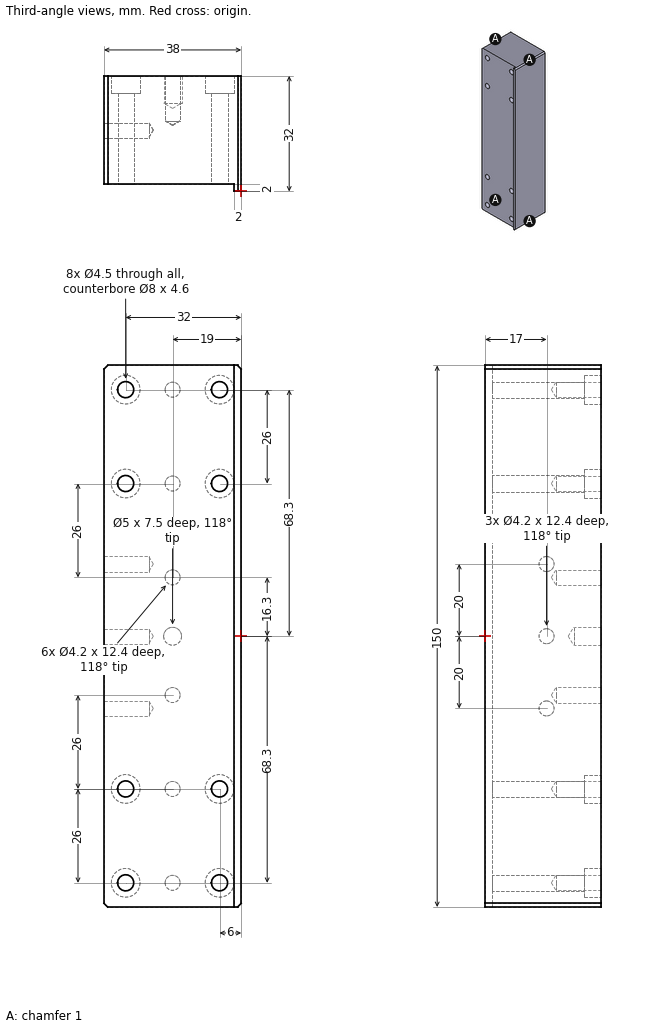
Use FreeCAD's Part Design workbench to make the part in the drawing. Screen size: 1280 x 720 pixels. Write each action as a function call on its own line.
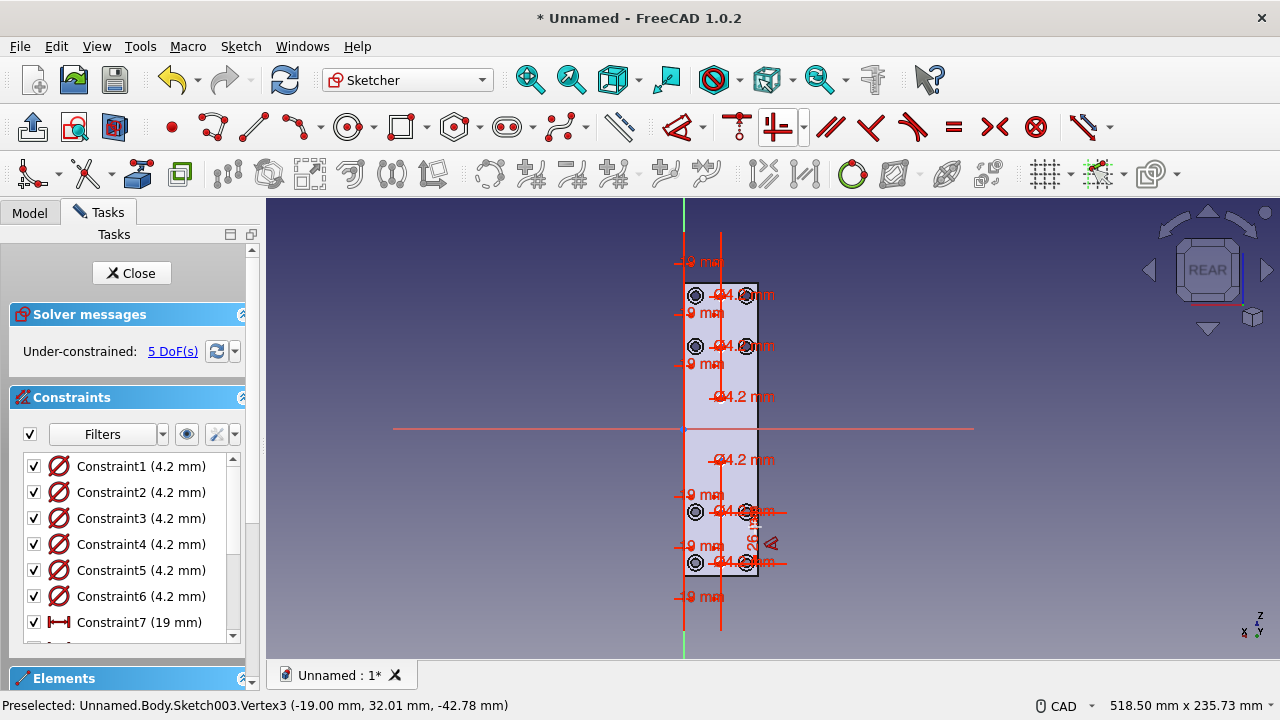
click(721, 399)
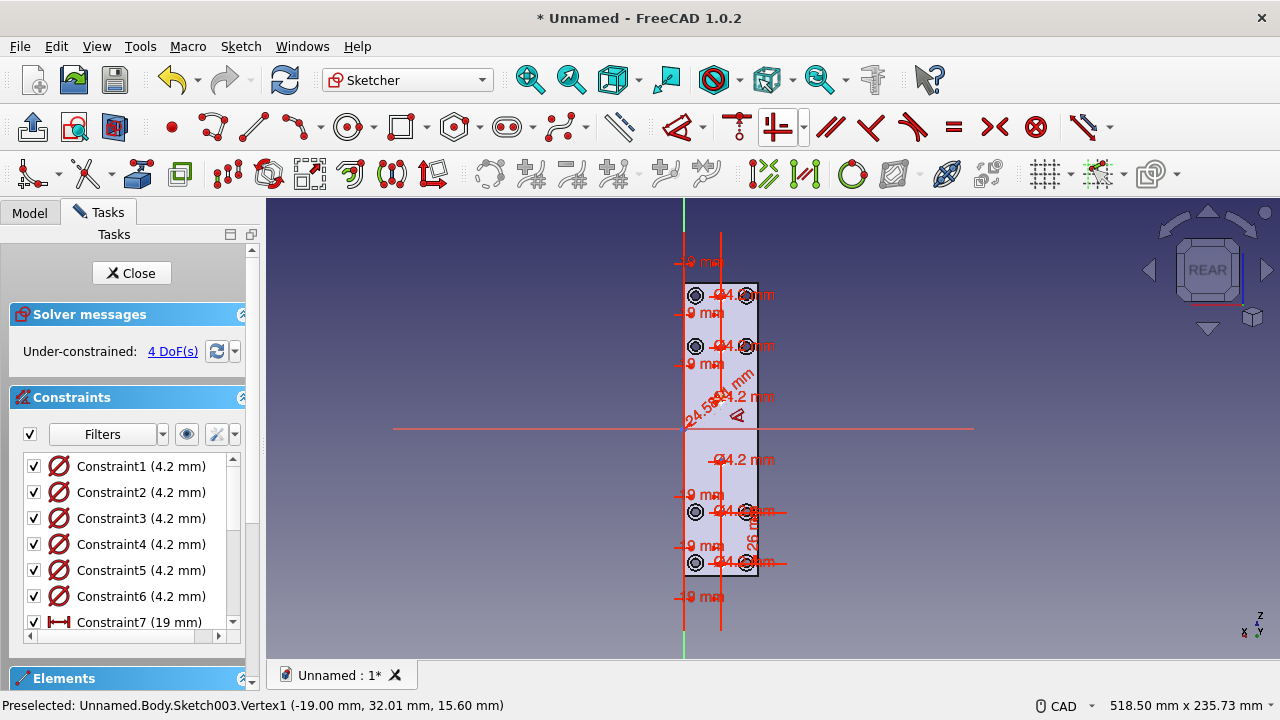
click(721, 348)
click(755, 385)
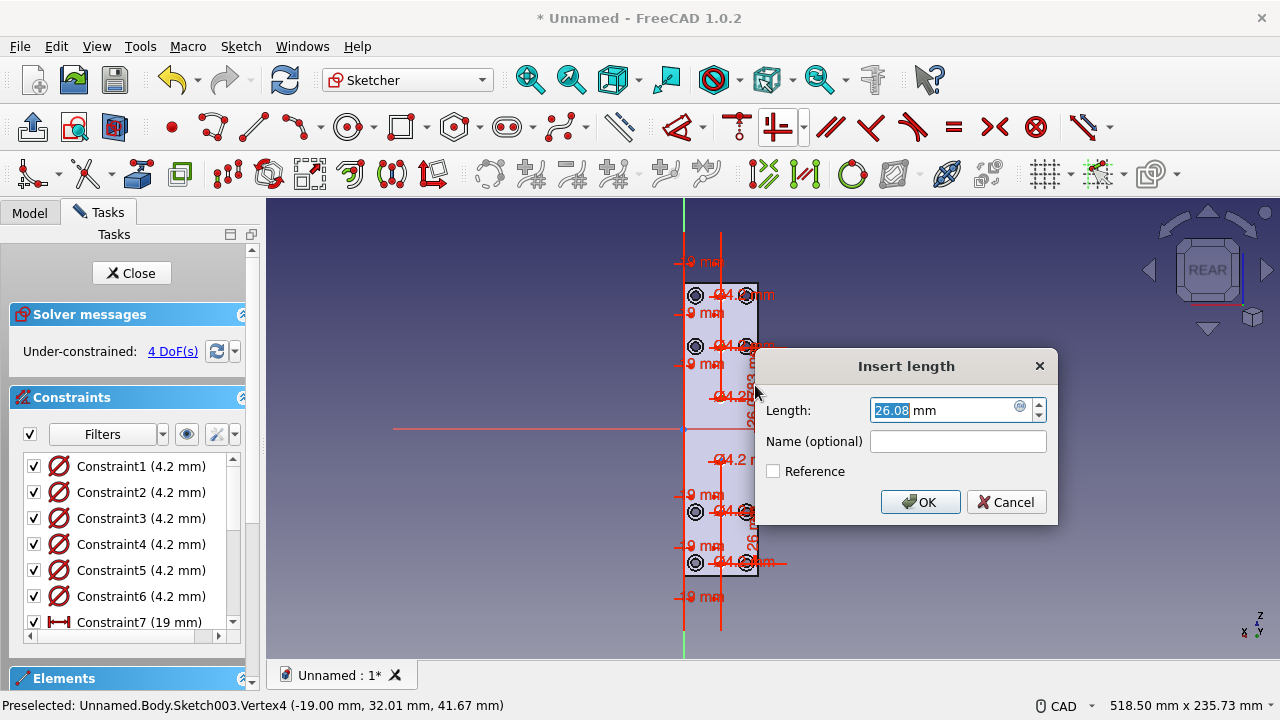
text(26)
key(Return)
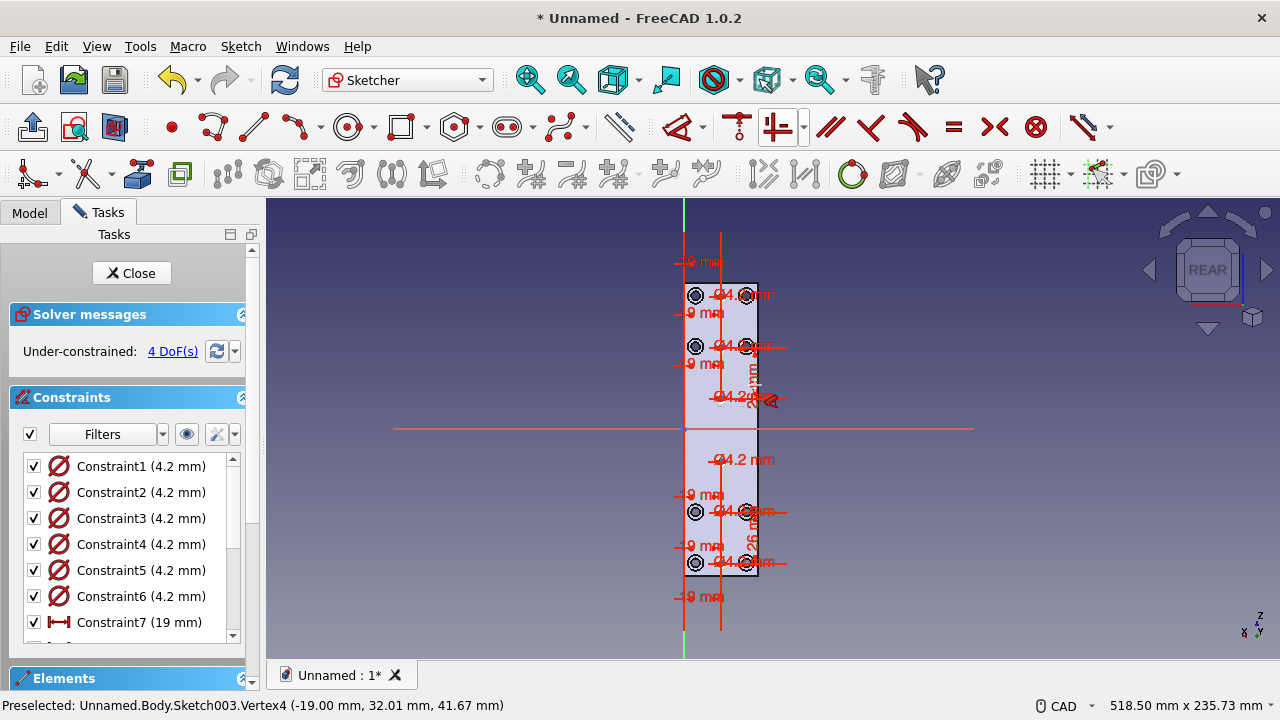
click(721, 348)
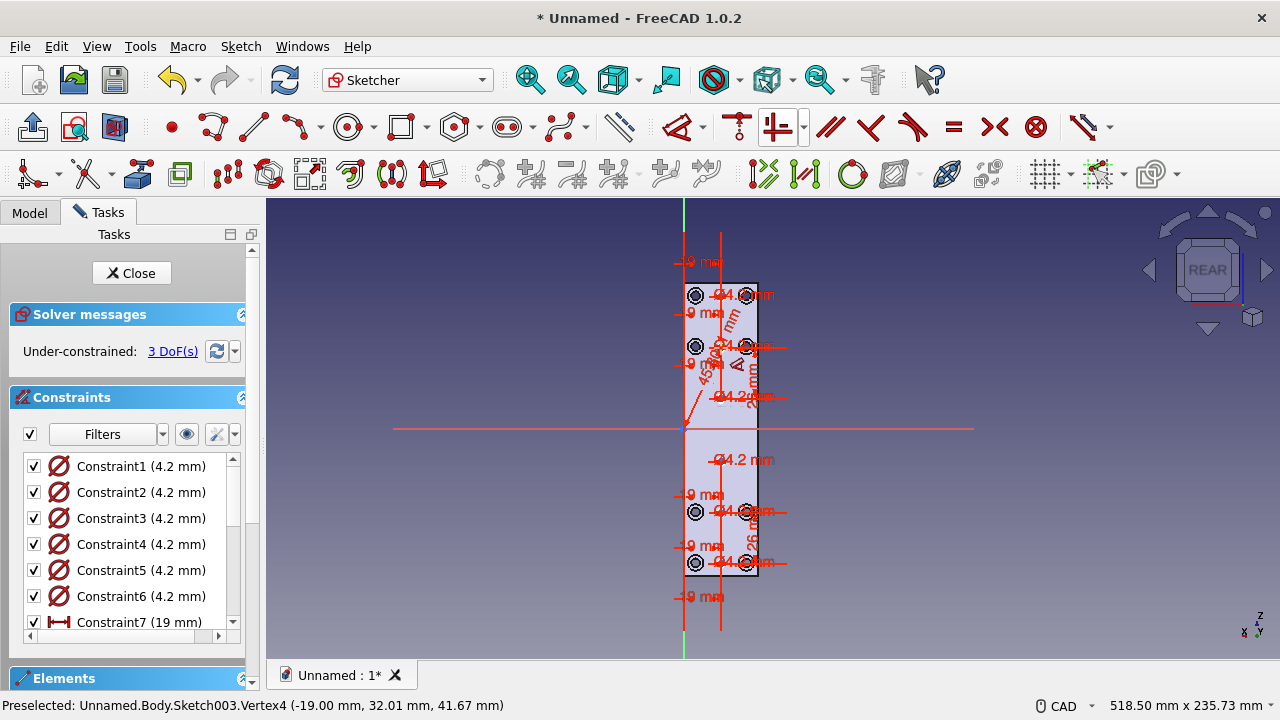
click(721, 297)
click(755, 334)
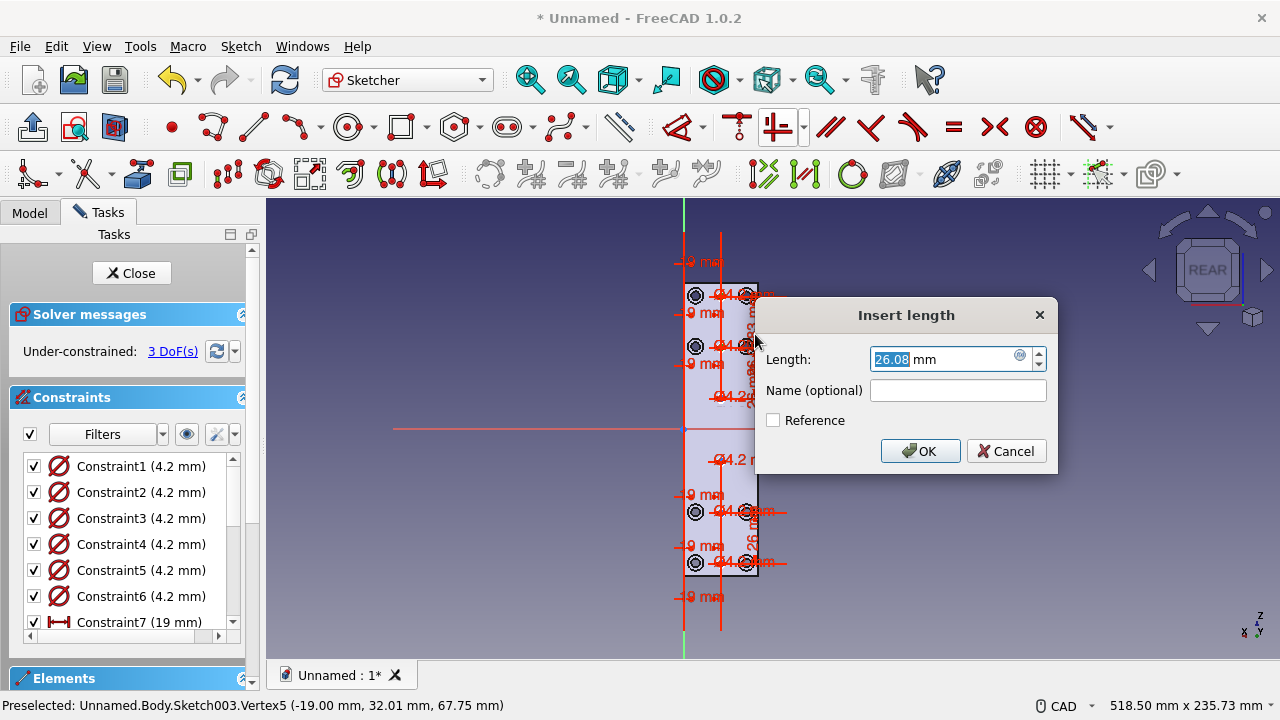
text(26)
key(Return)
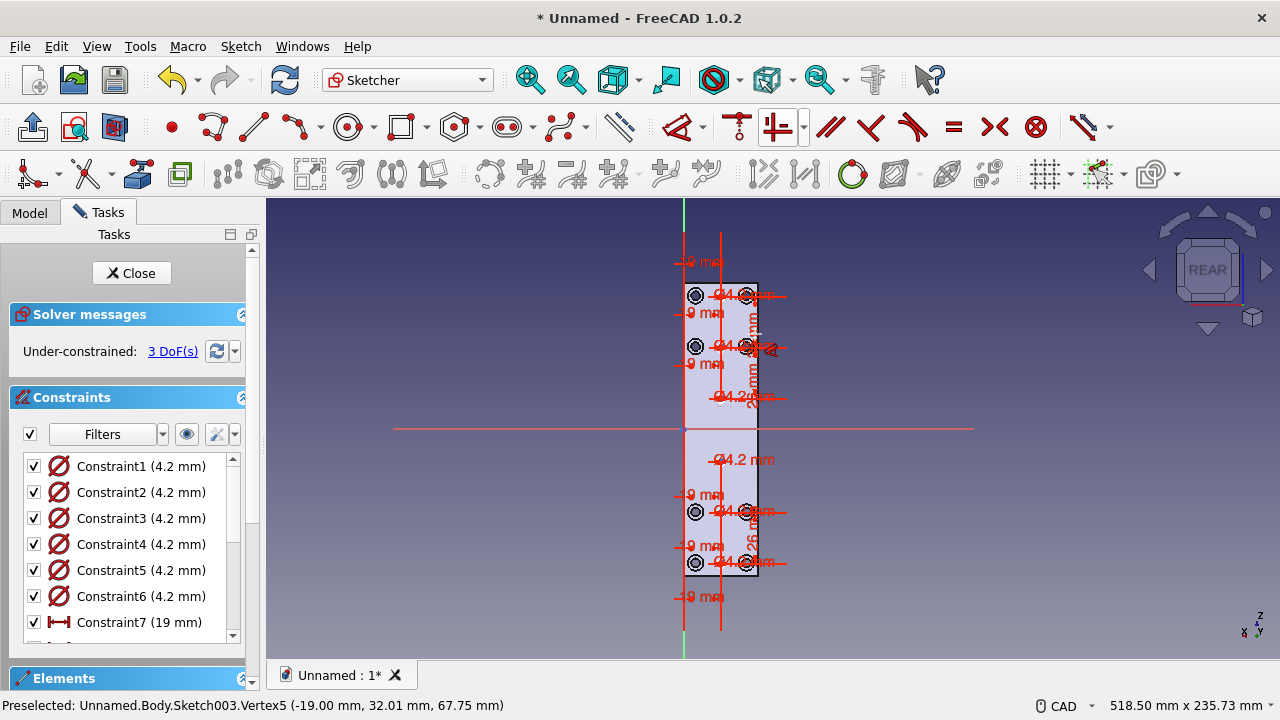
click(721, 513)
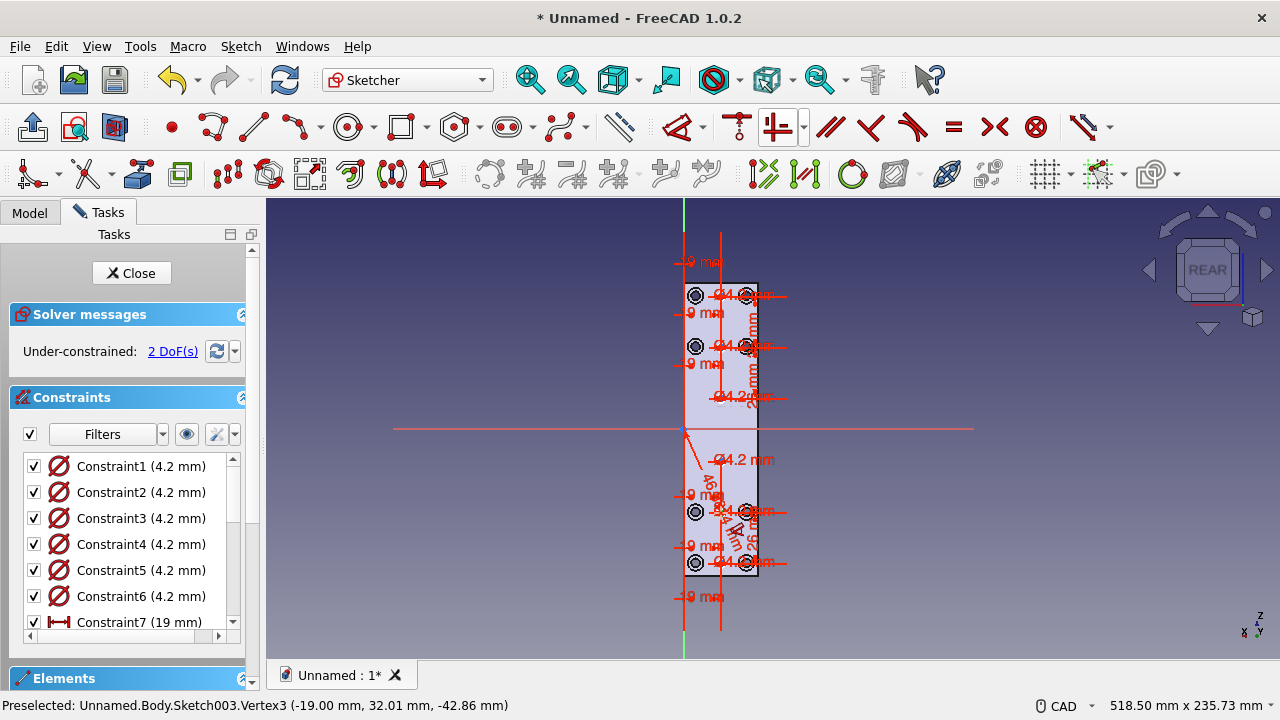
click(721, 462)
click(755, 476)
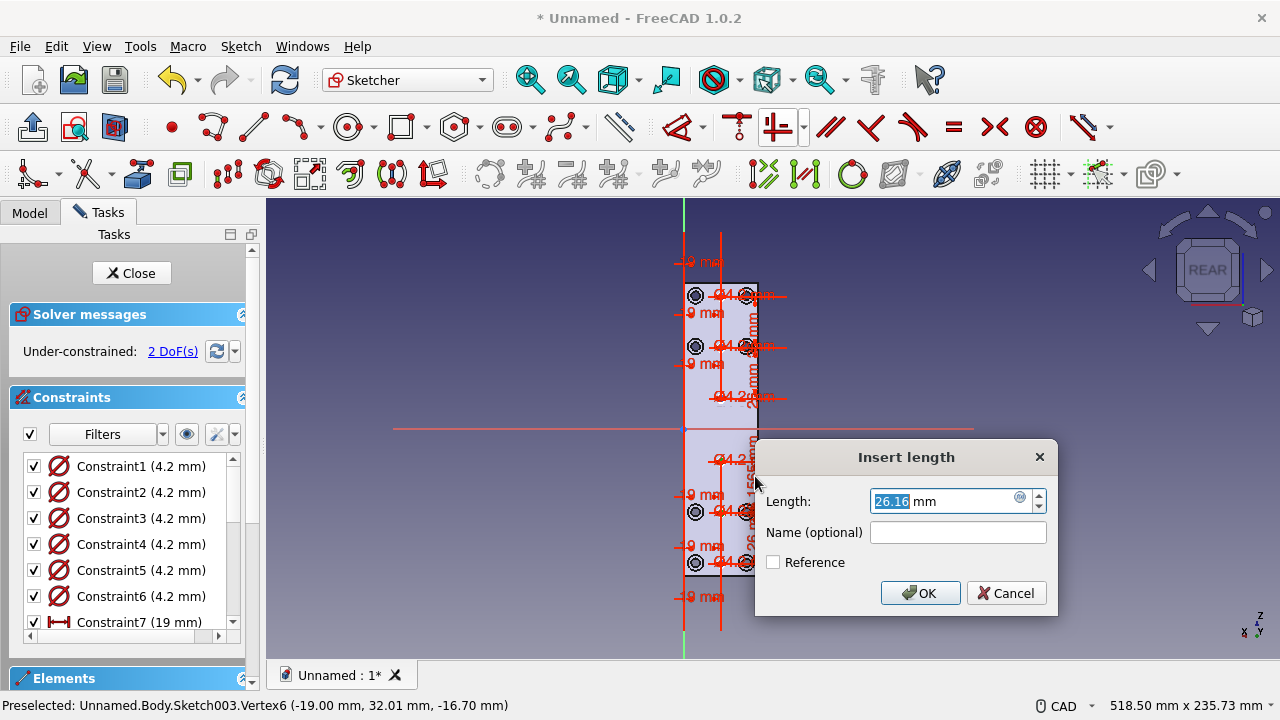
text(26)
key(Return)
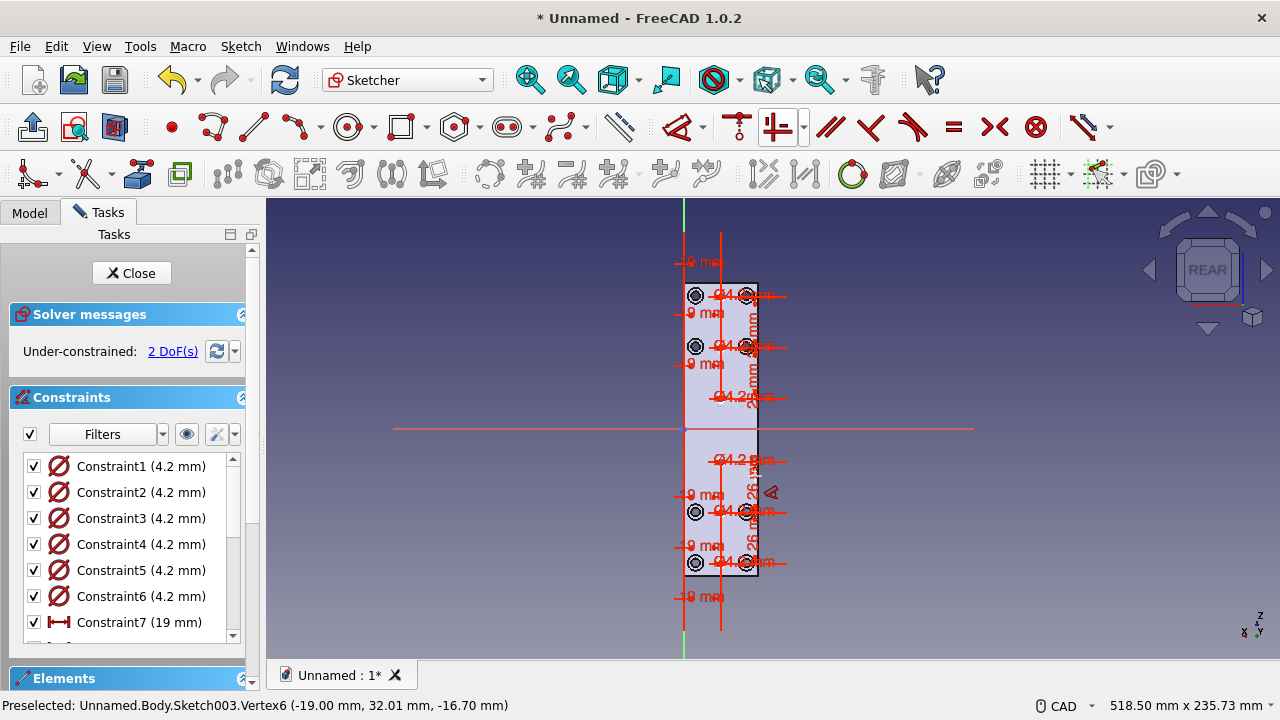
scroll(721, 399, up, 2)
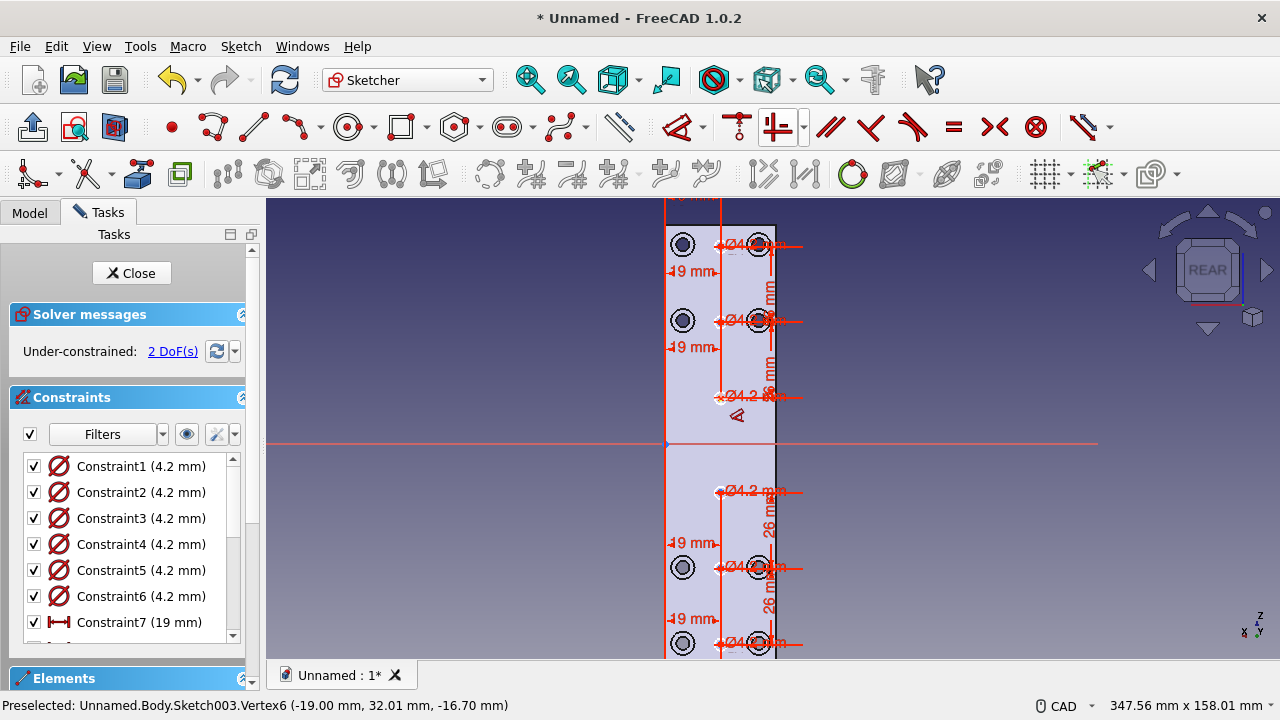
click(721, 398)
click(631, 421)